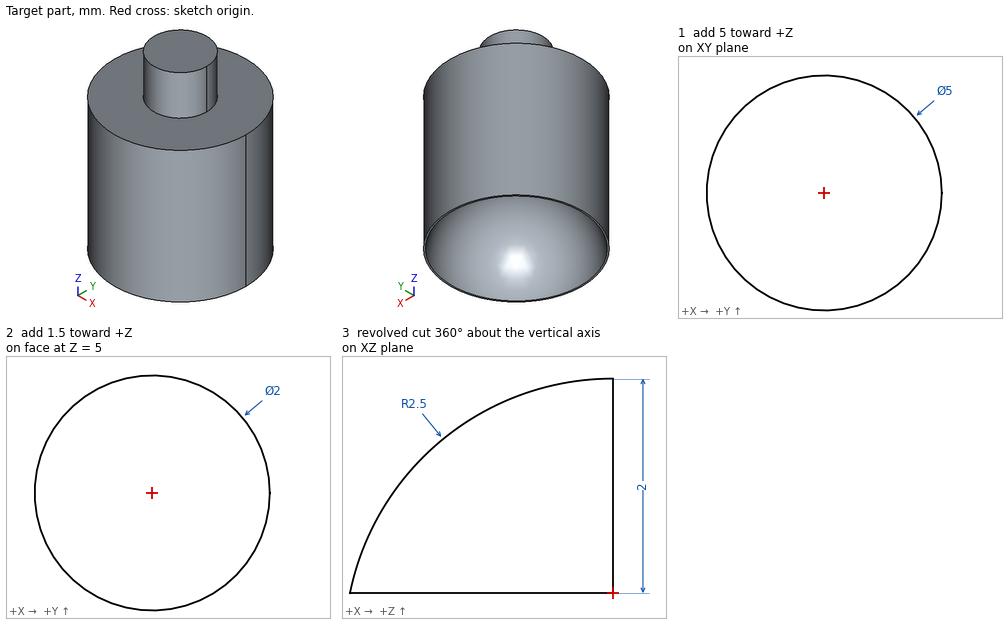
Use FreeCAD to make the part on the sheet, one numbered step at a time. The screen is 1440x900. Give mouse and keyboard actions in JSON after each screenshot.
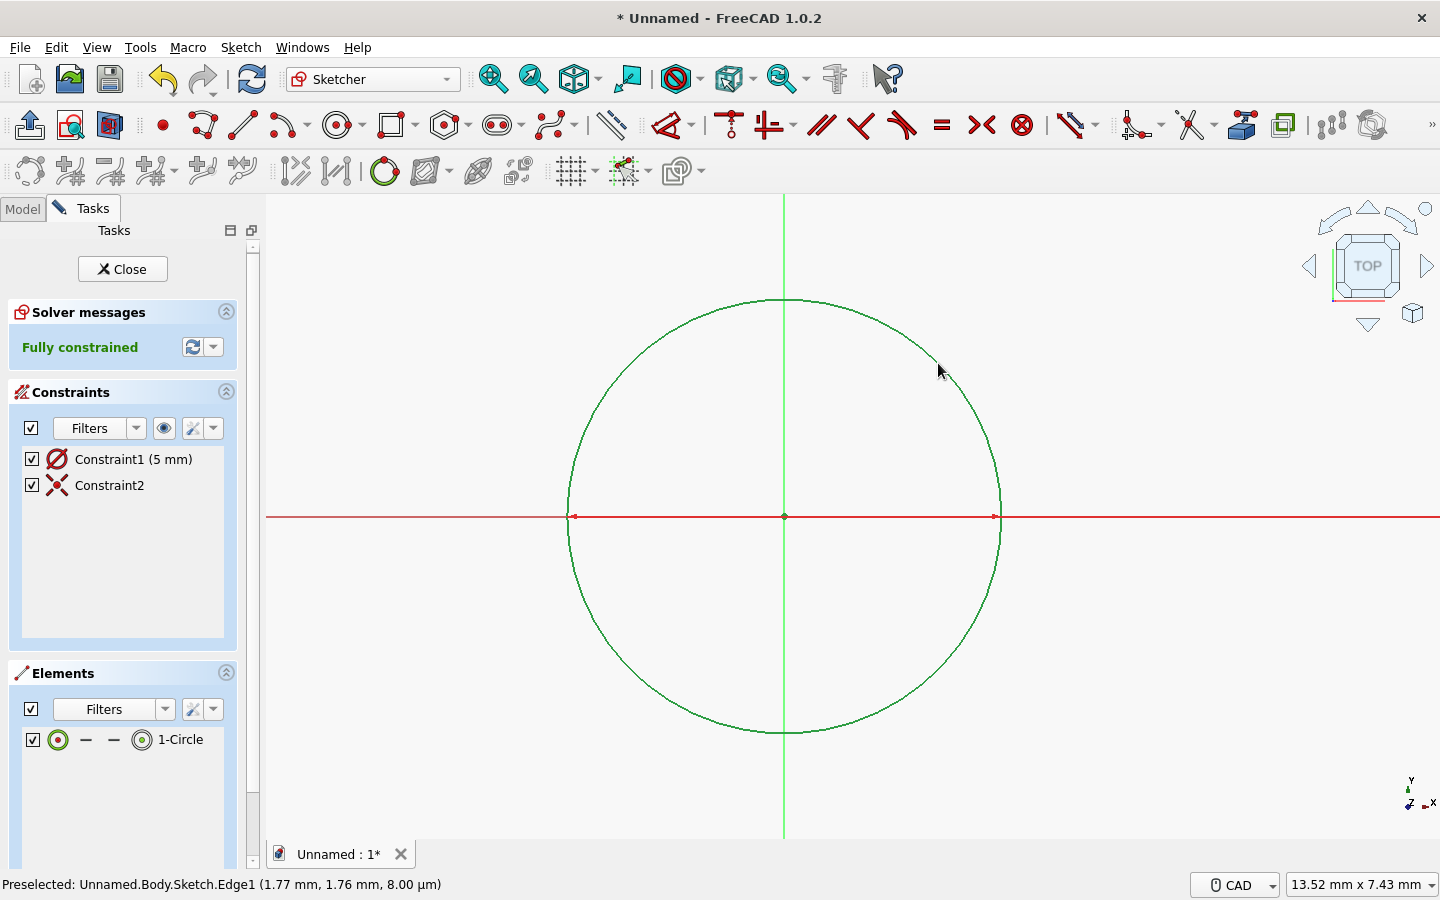
{"action": "left_click", "coordinate": [123, 269]}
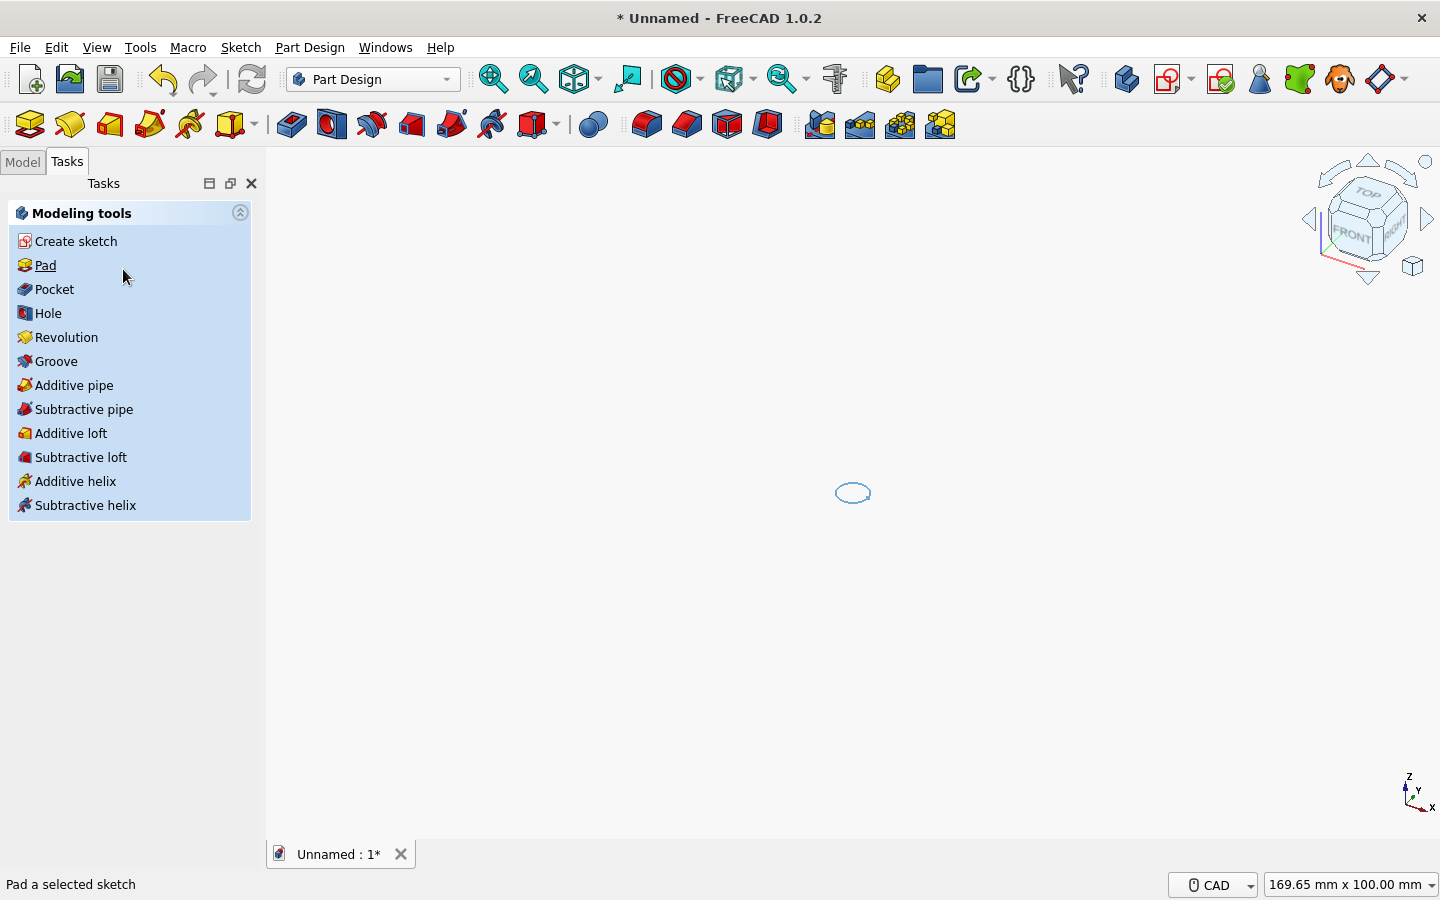
{"action": "left_click", "coordinate": [30, 124]}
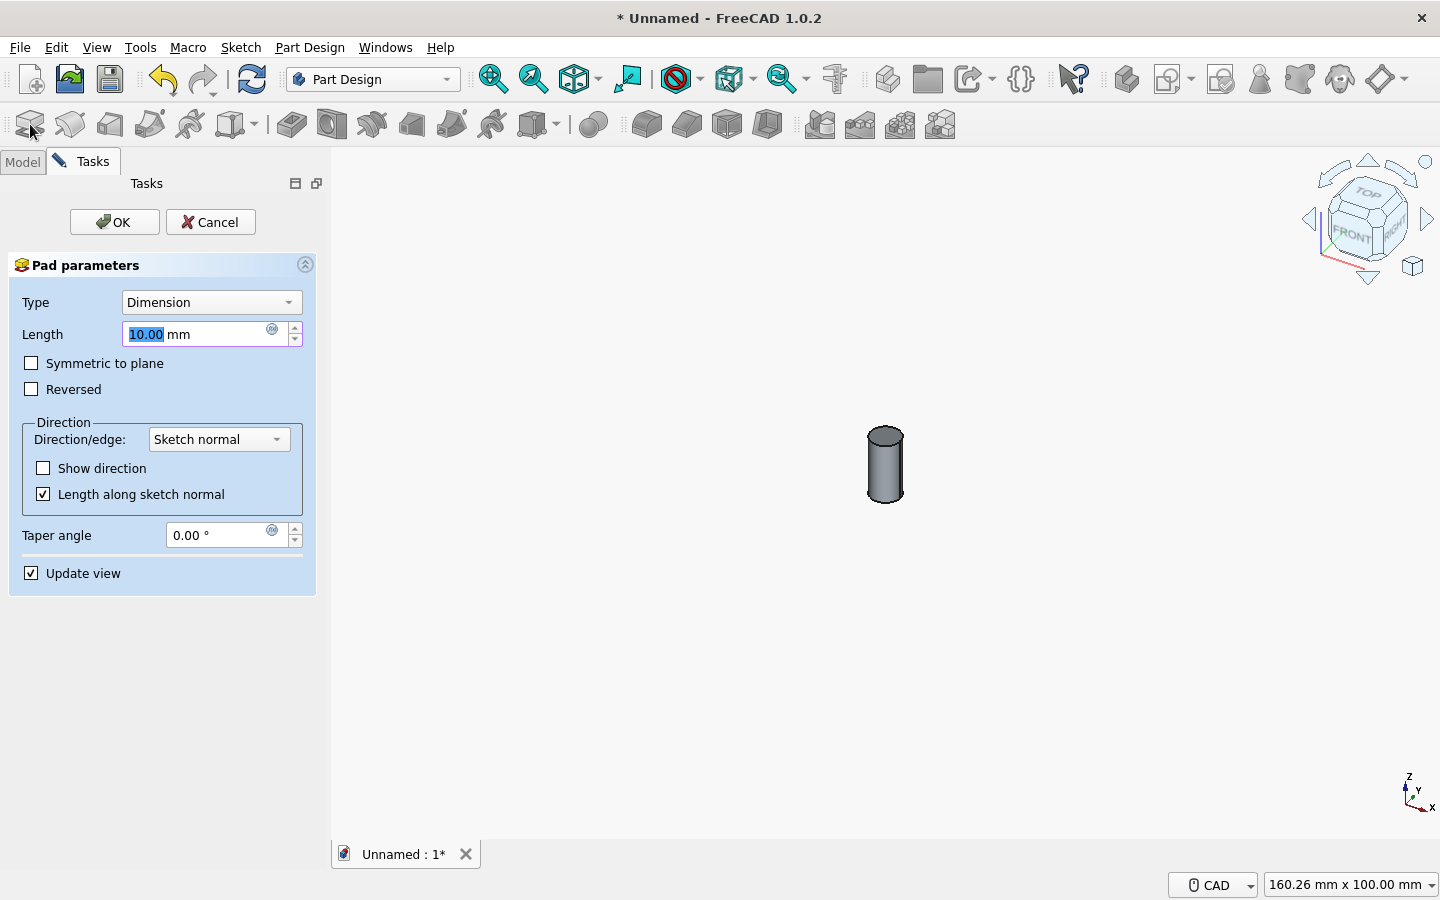
{"action": "type", "text": "5"}
{"action": "key", "text": "Tab"}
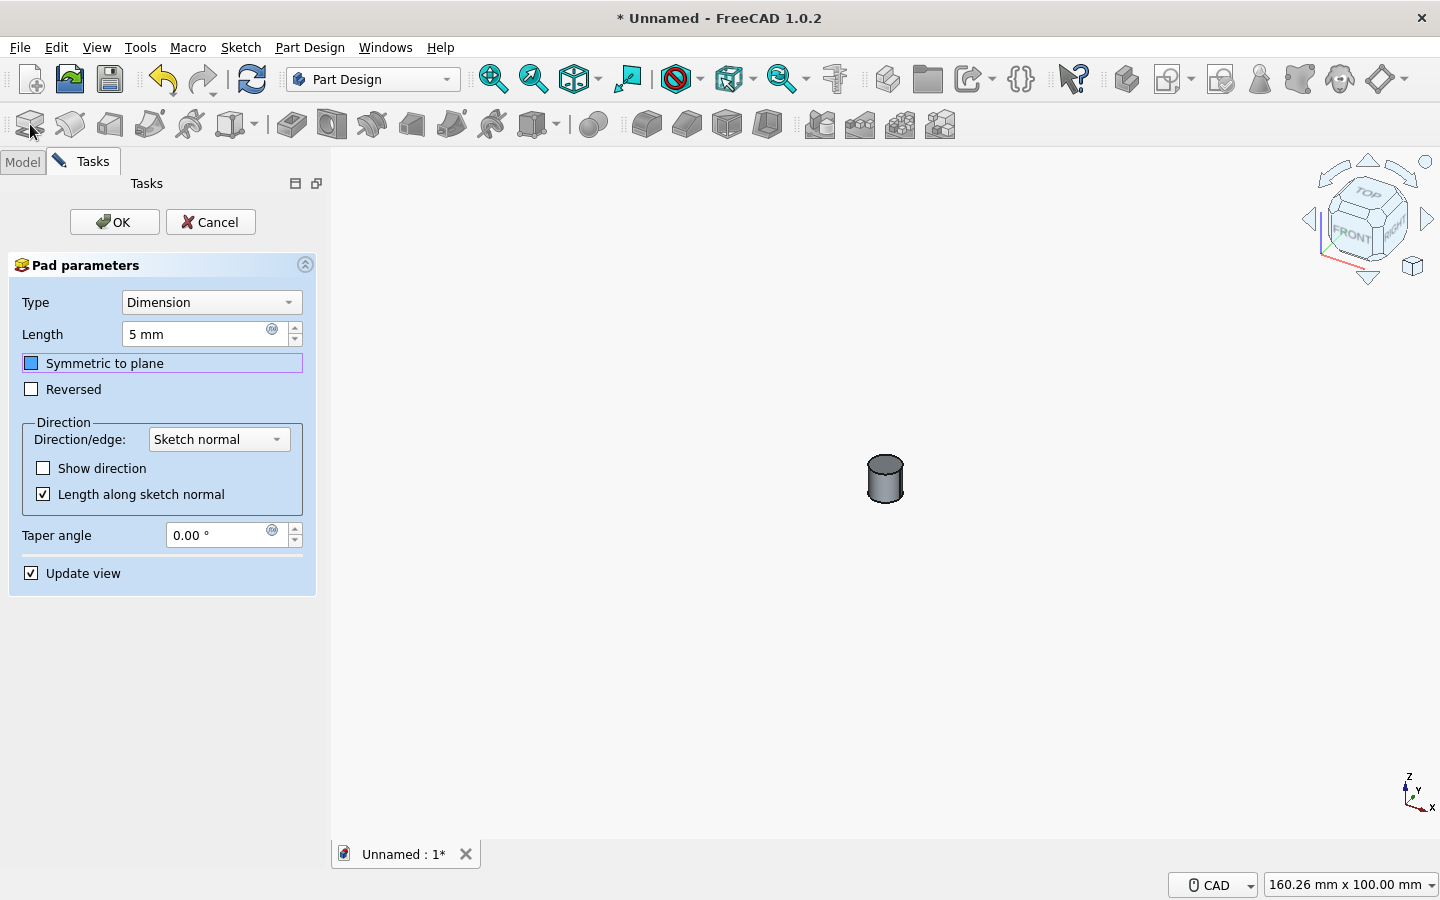
{"action": "left_click", "coordinate": [115, 222]}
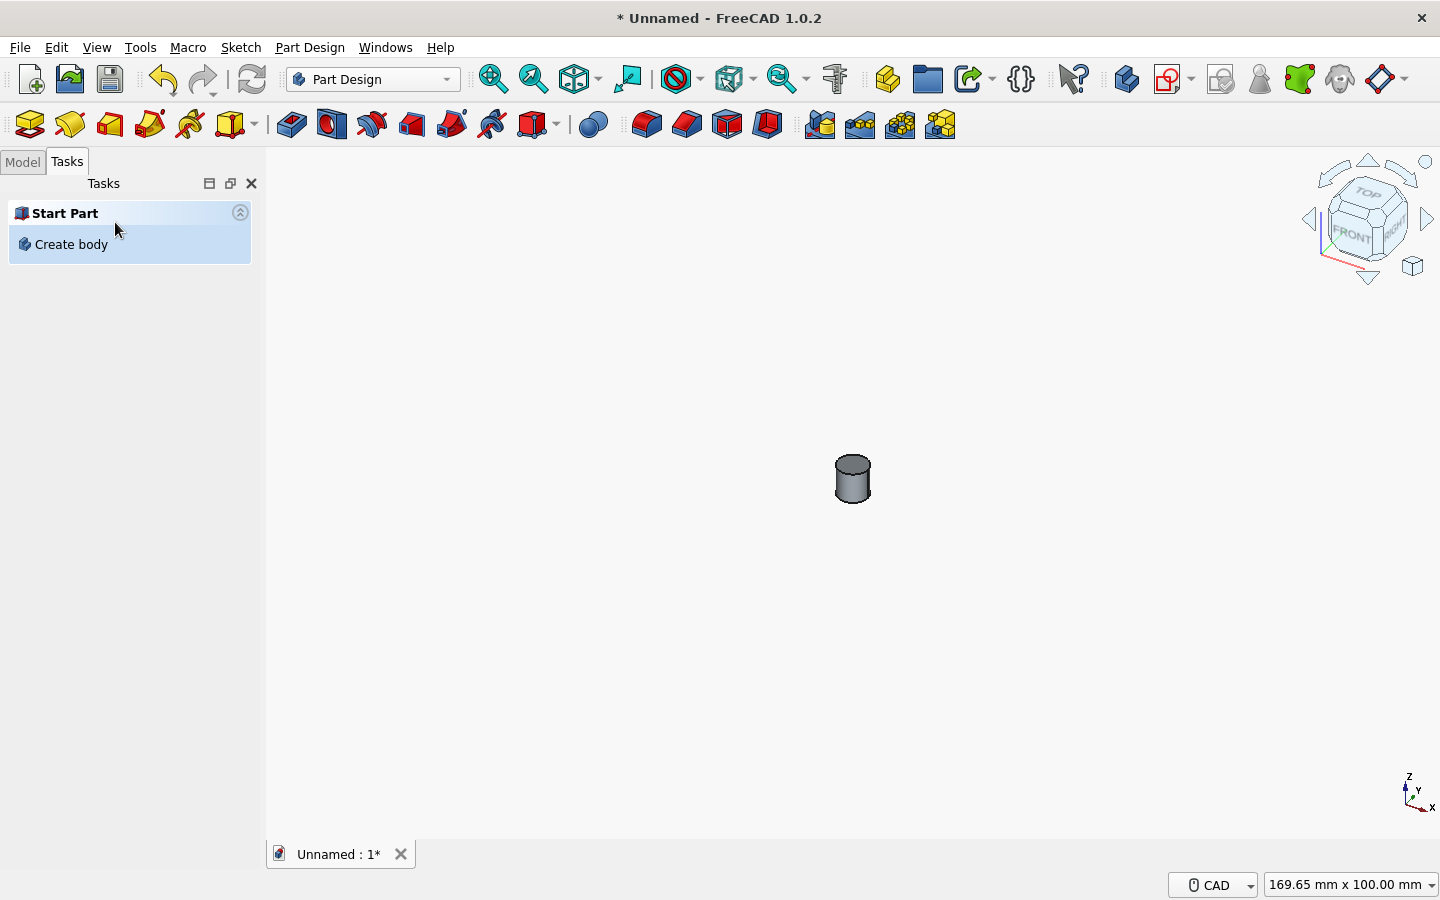
{"action": "left_click", "coordinate": [494, 80]}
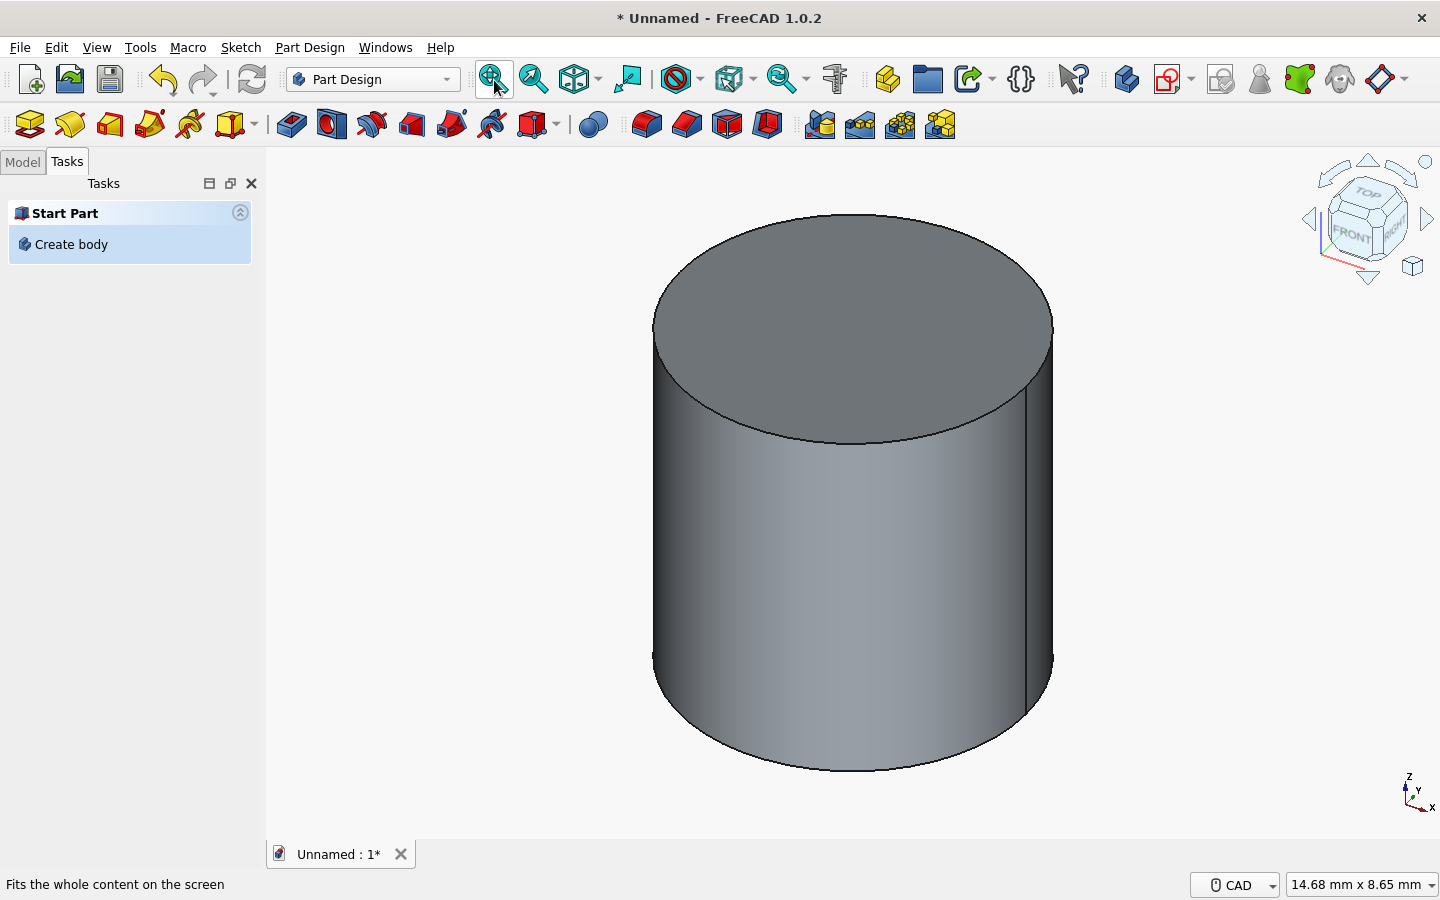
{"action": "left_click", "coordinate": [853, 328]}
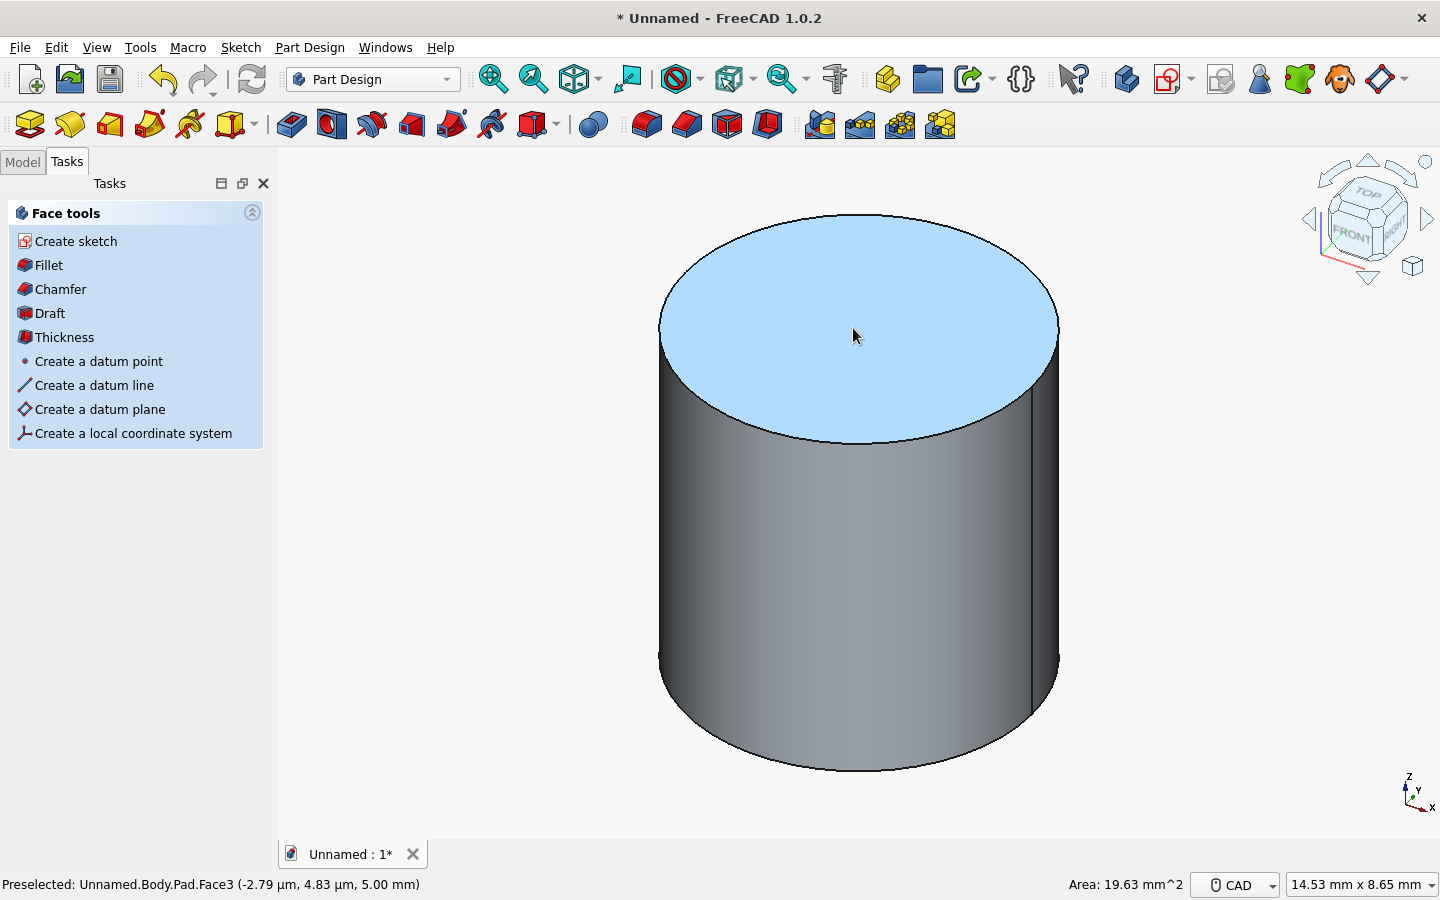
{"action": "left_click", "coordinate": [1168, 80]}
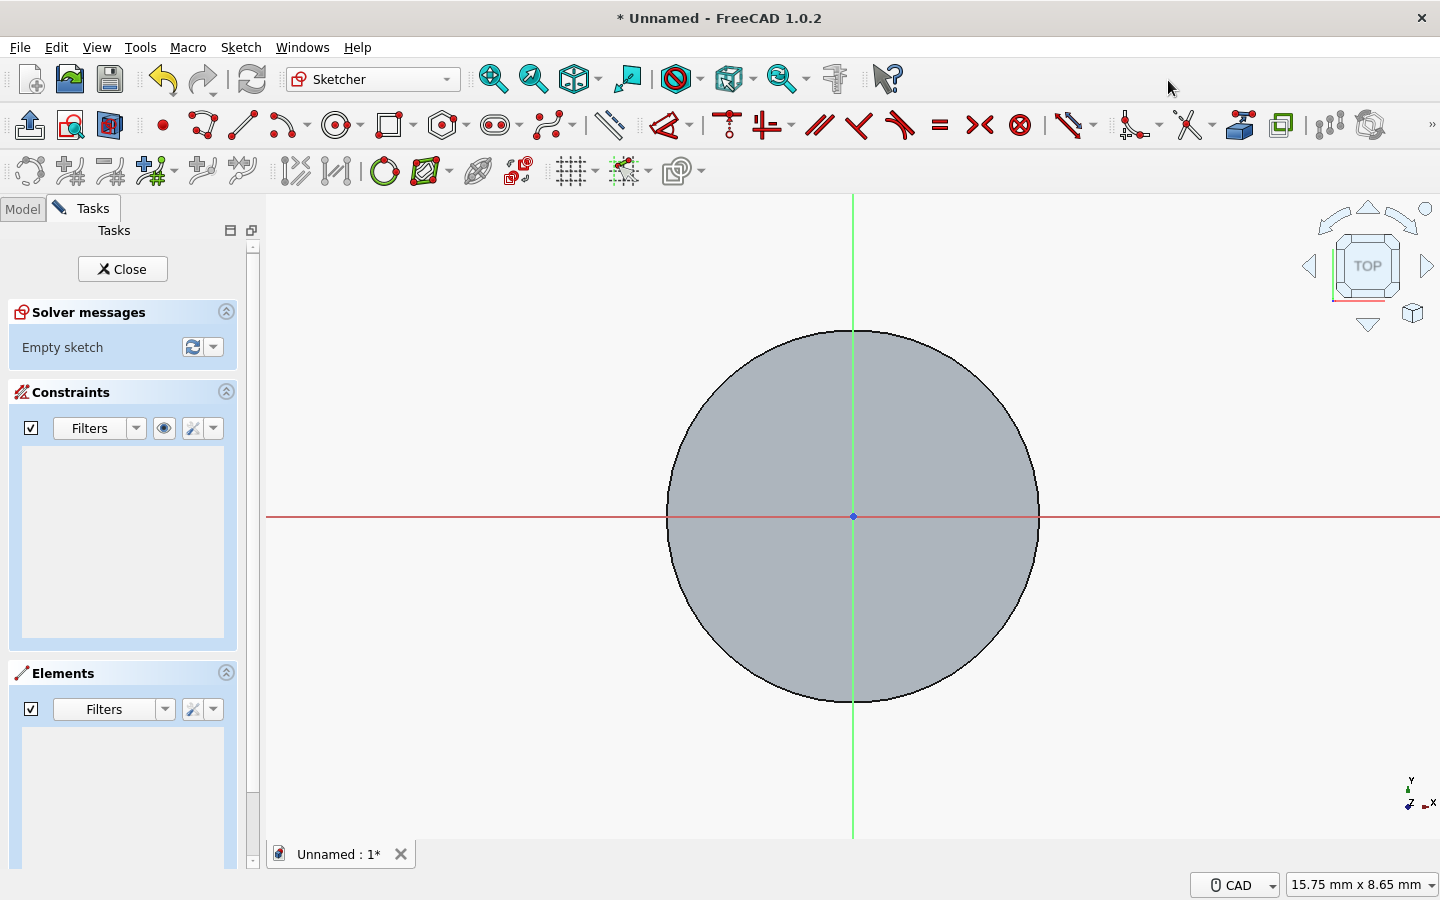
{"action": "scroll", "coordinate": [893, 516], "scroll_direction": "up", "scroll_amount": 5}